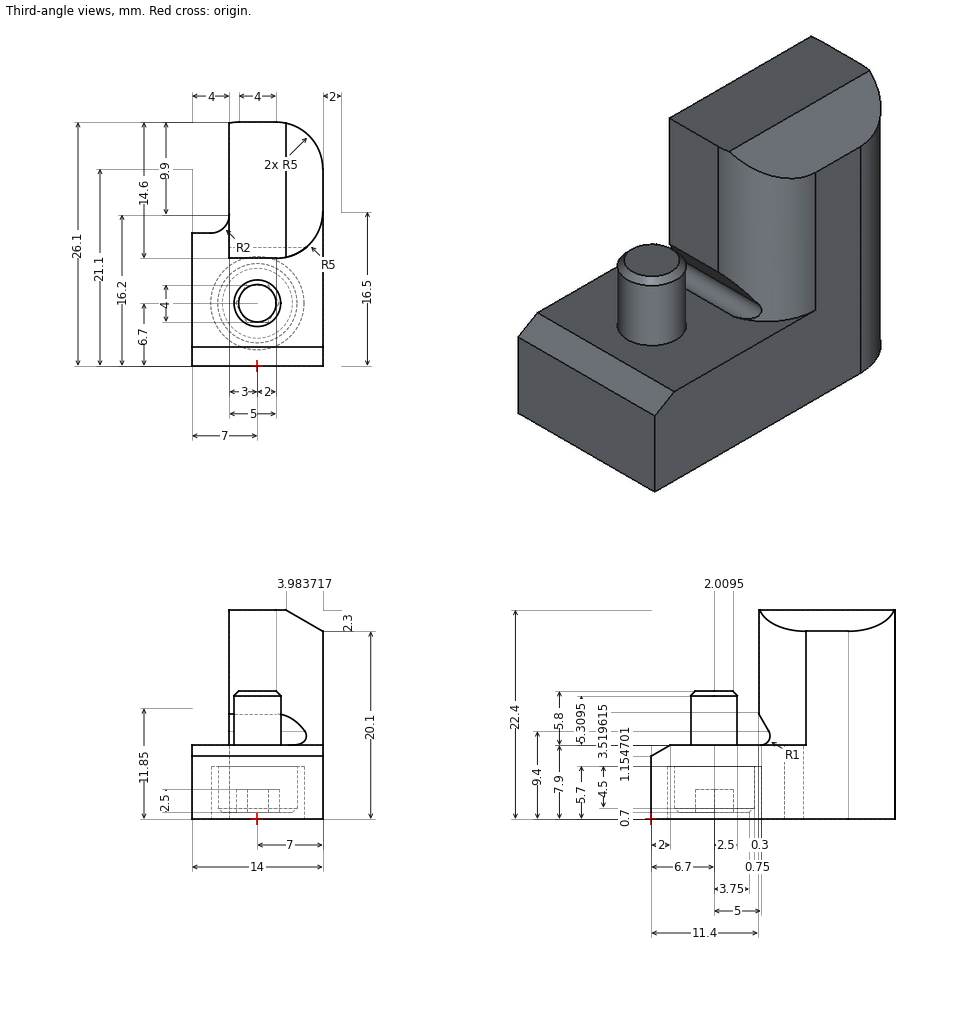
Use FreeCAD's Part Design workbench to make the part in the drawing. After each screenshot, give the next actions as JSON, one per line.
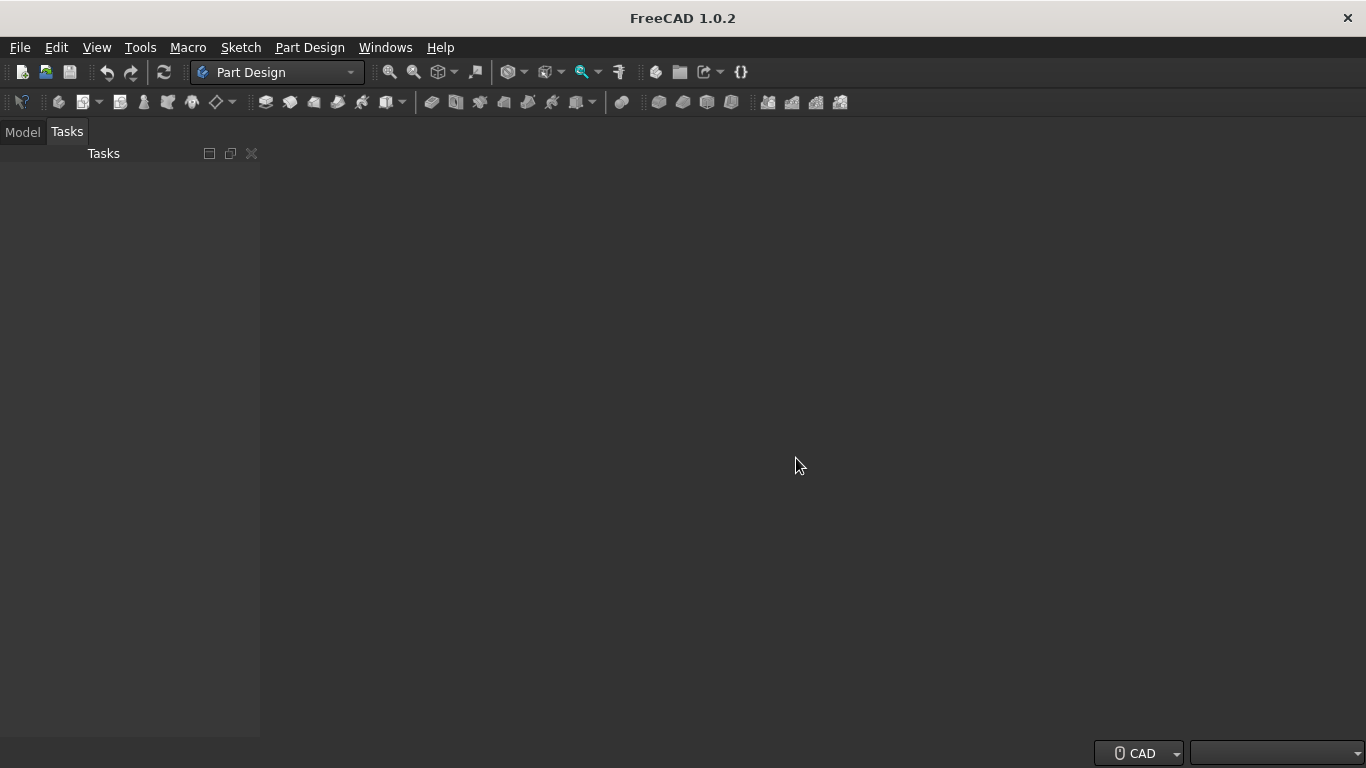
{"action": "left_click", "coordinate": [22, 72]}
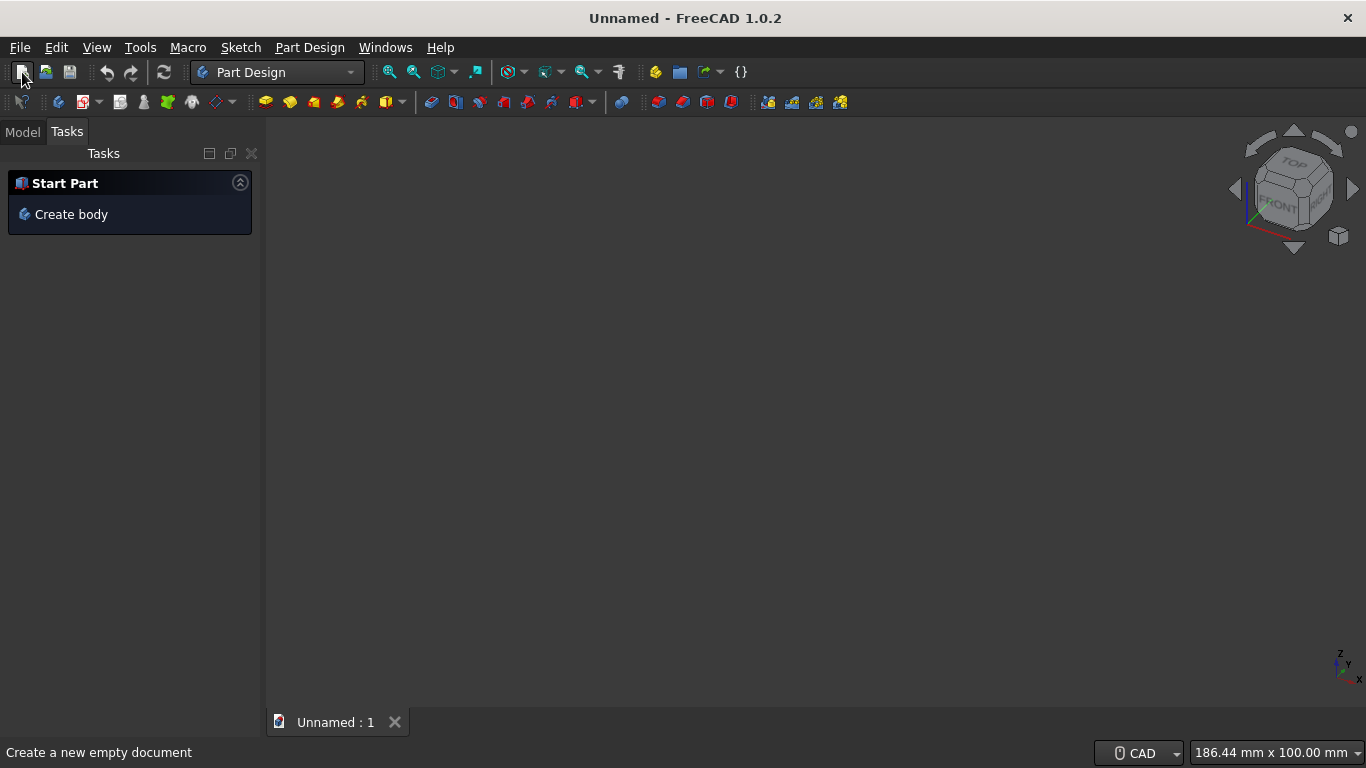
{"action": "left_click", "coordinate": [84, 102]}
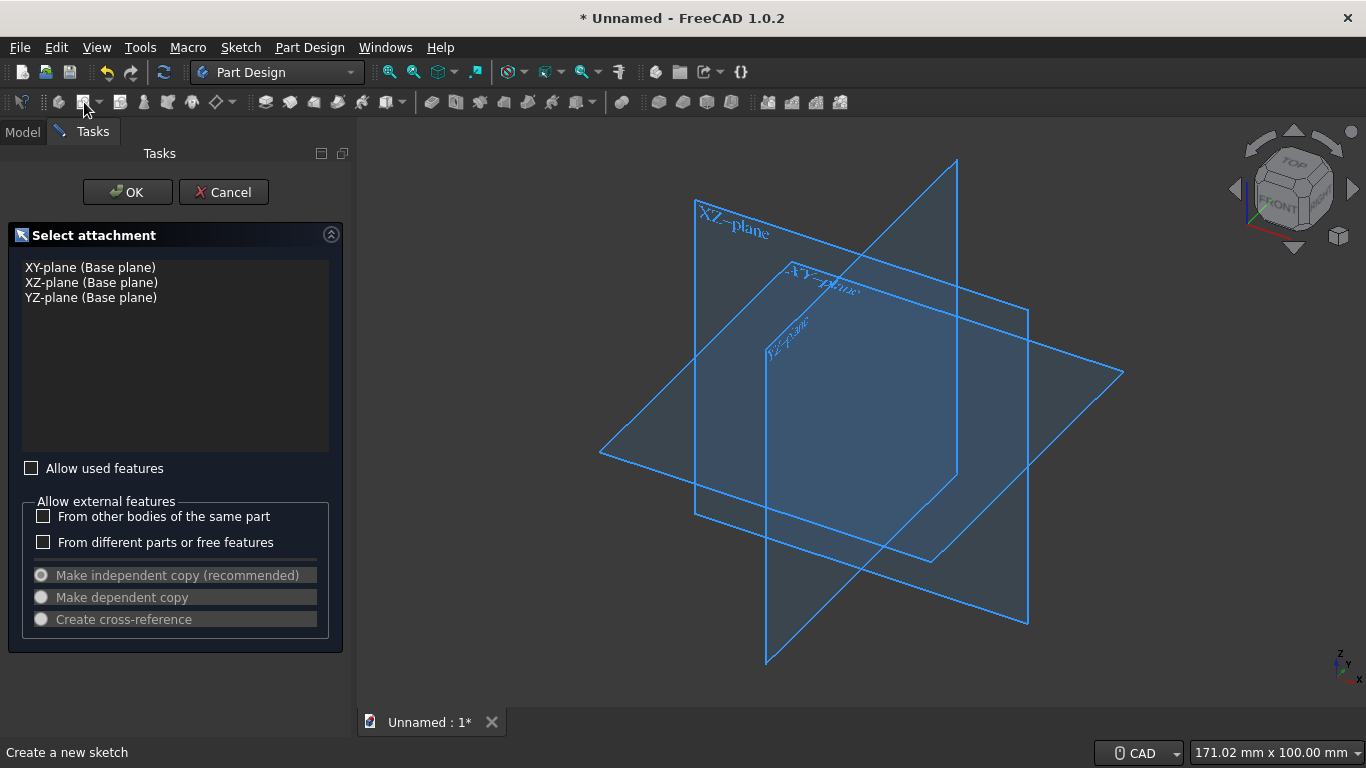
{"action": "left_click", "coordinate": [82, 268]}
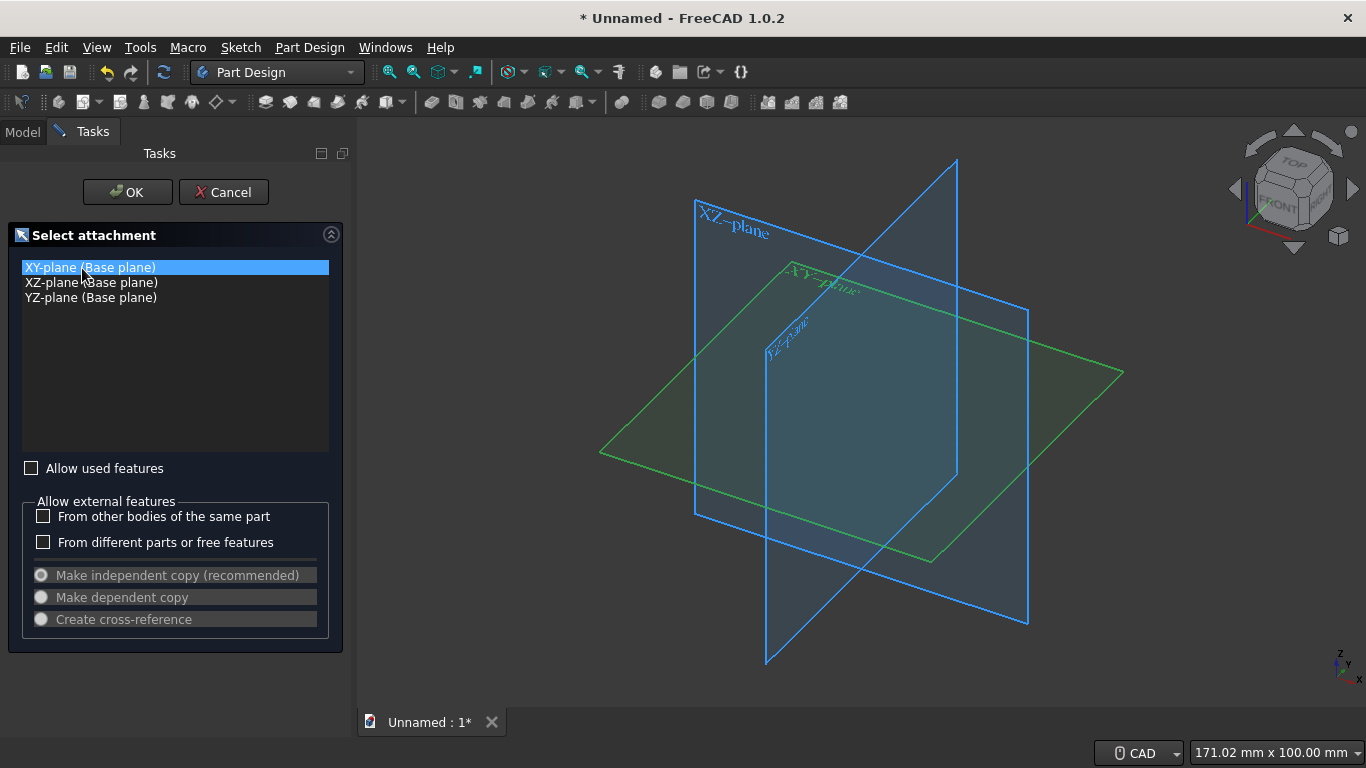
{"action": "left_click", "coordinate": [128, 192]}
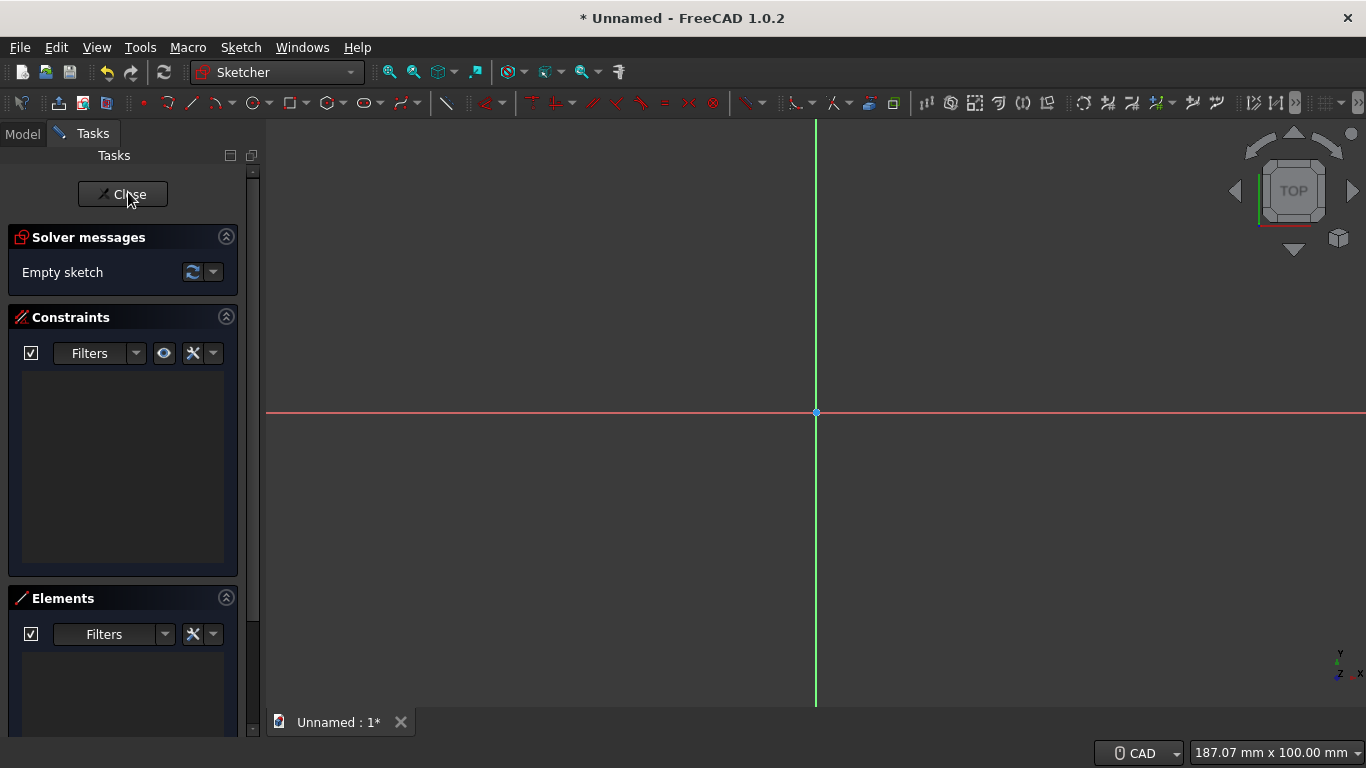
{"action": "scroll", "coordinate": [872, 274], "scroll_direction": "up", "scroll_amount": 4}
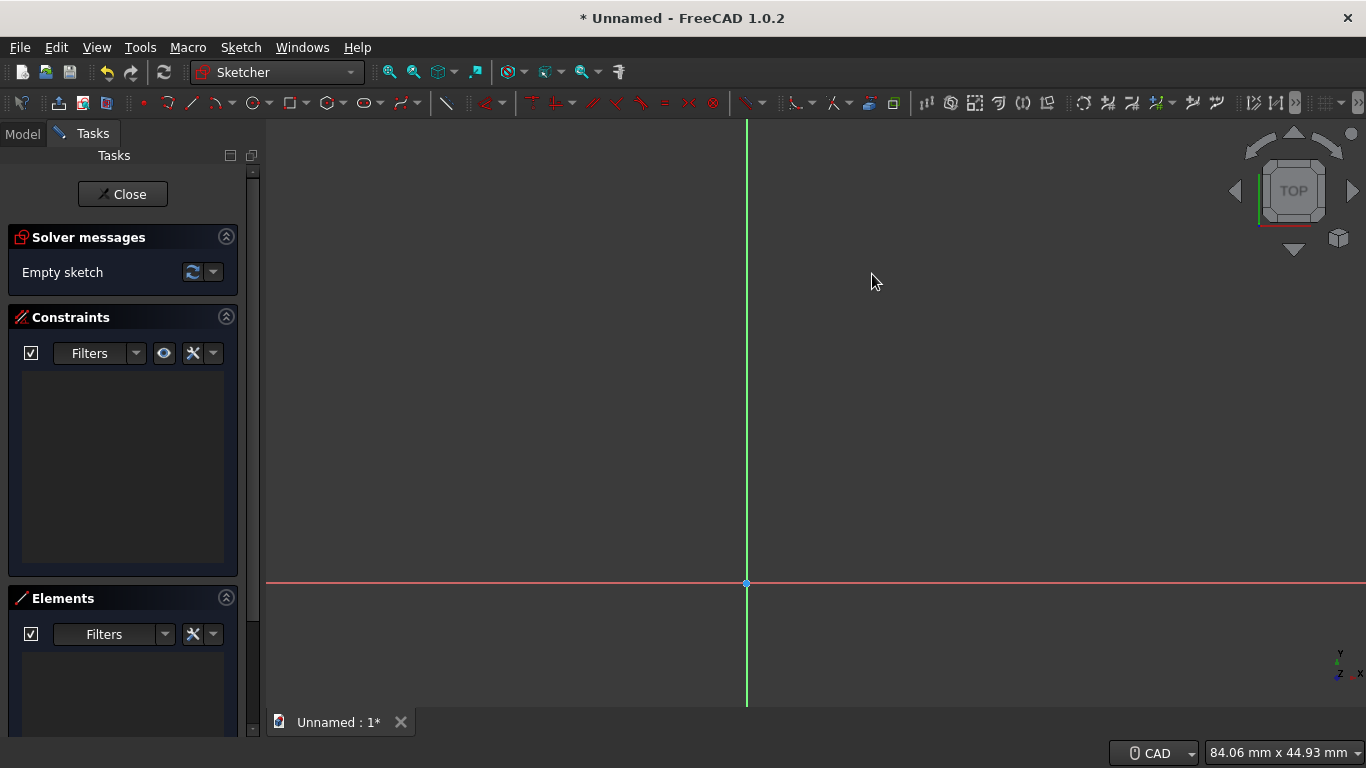
{"action": "left_click", "coordinate": [168, 104]}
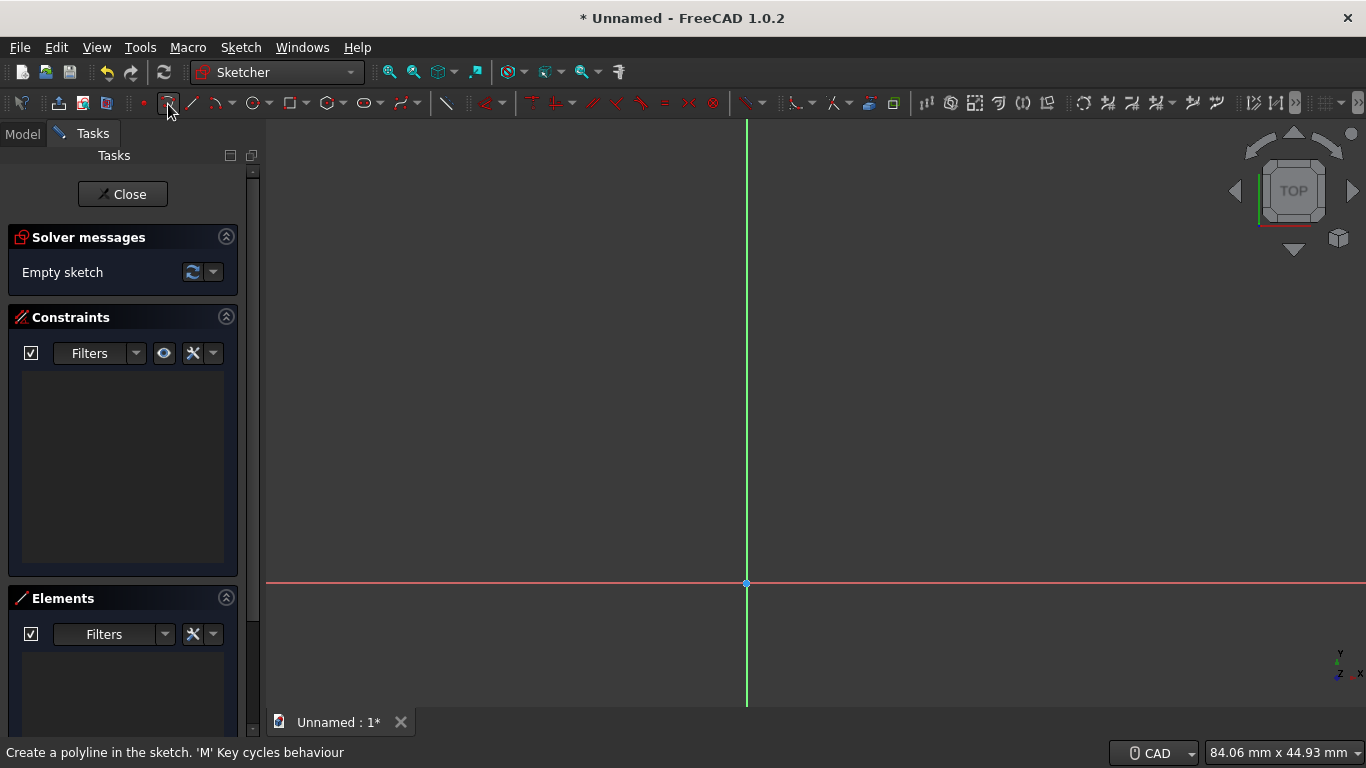
{"action": "left_click", "coordinate": [655, 307]}
{"action": "left_click", "coordinate": [655, 583]}
{"action": "left_click", "coordinate": [838, 574]}
{"action": "left_click", "coordinate": [838, 307]}
{"action": "right_click", "coordinate": [838, 307]}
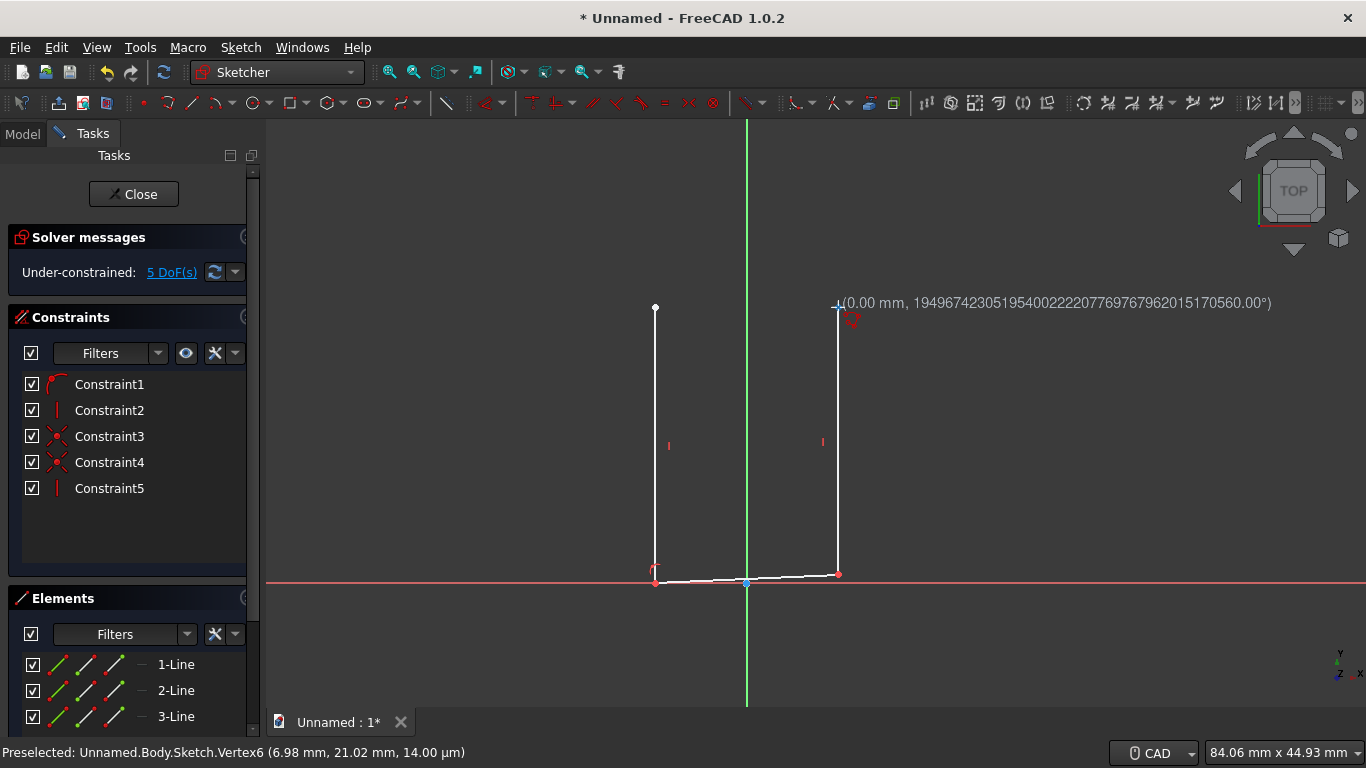
{"action": "left_click", "coordinate": [192, 104]}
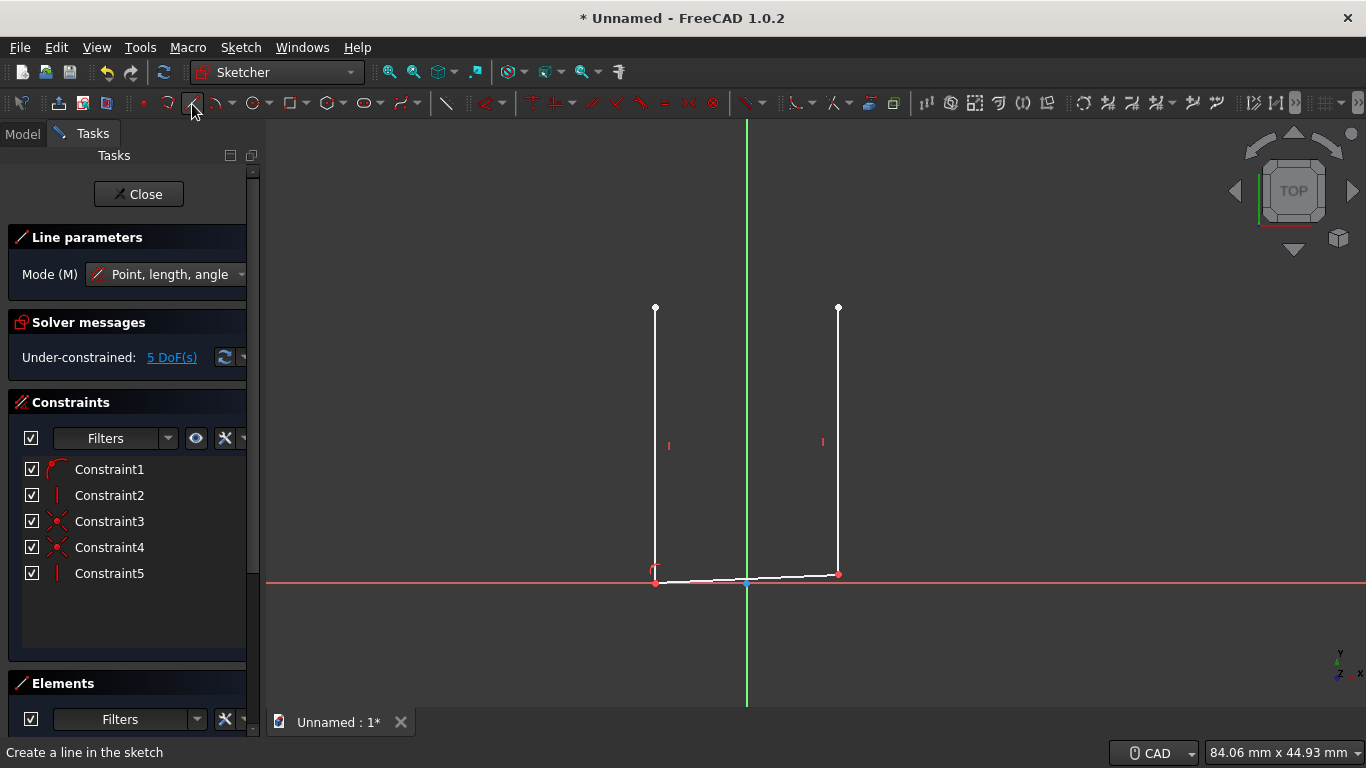
{"action": "left_click", "coordinate": [773, 241]}
{"action": "left_click", "coordinate": [721, 241]}